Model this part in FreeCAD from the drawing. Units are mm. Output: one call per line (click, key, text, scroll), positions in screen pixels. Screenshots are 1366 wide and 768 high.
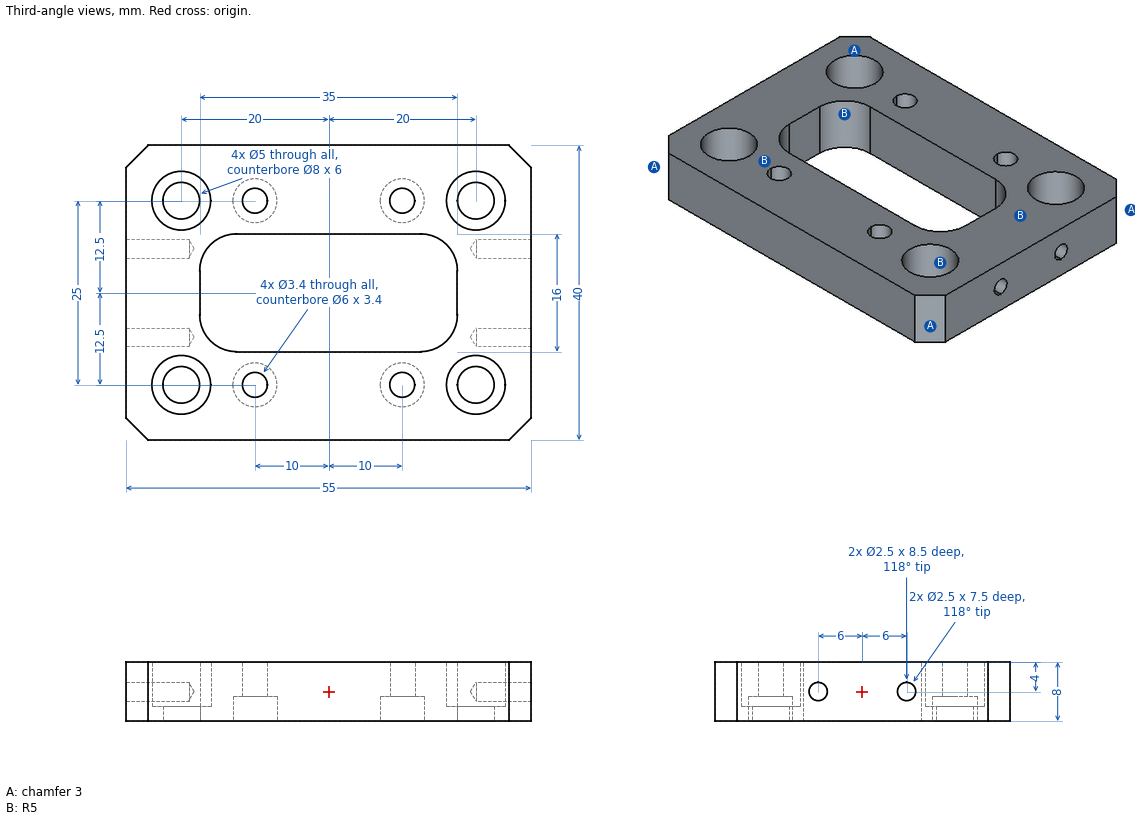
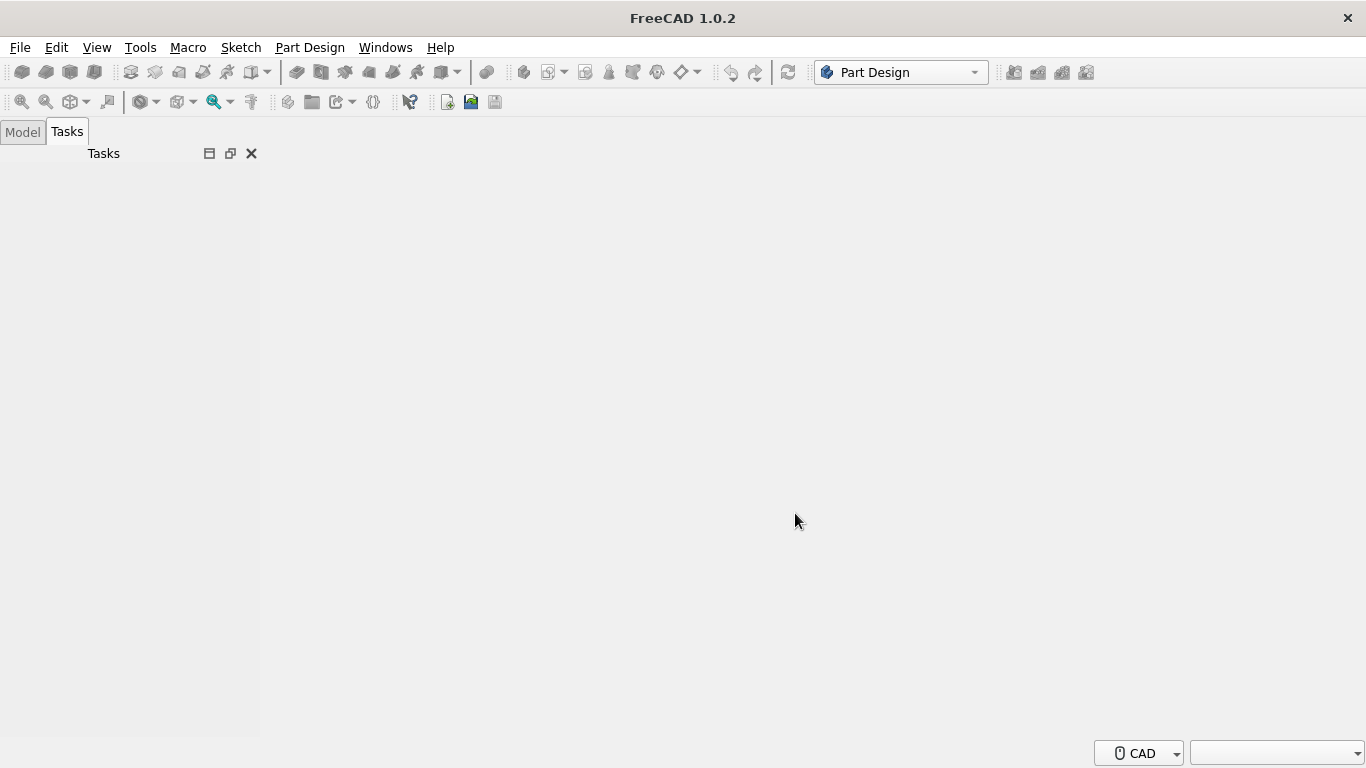
click(448, 102)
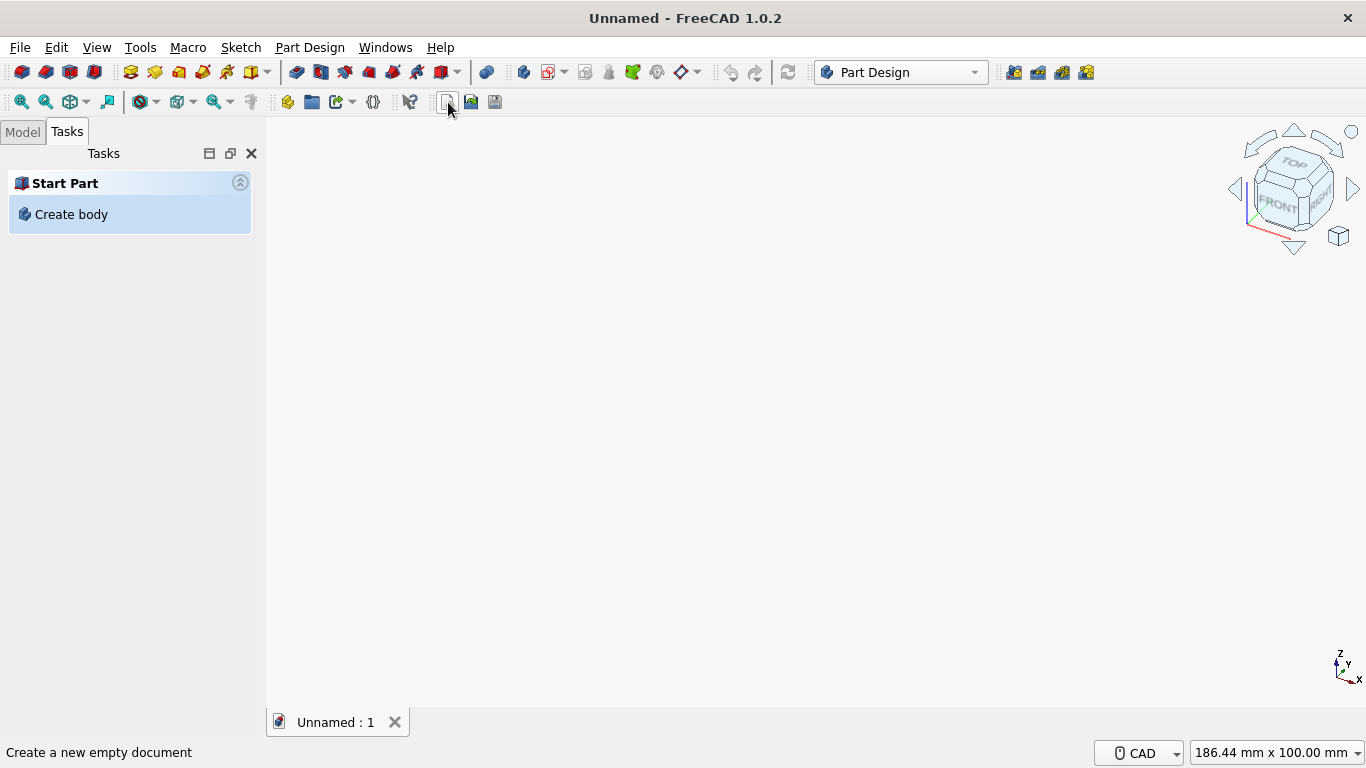
click(524, 72)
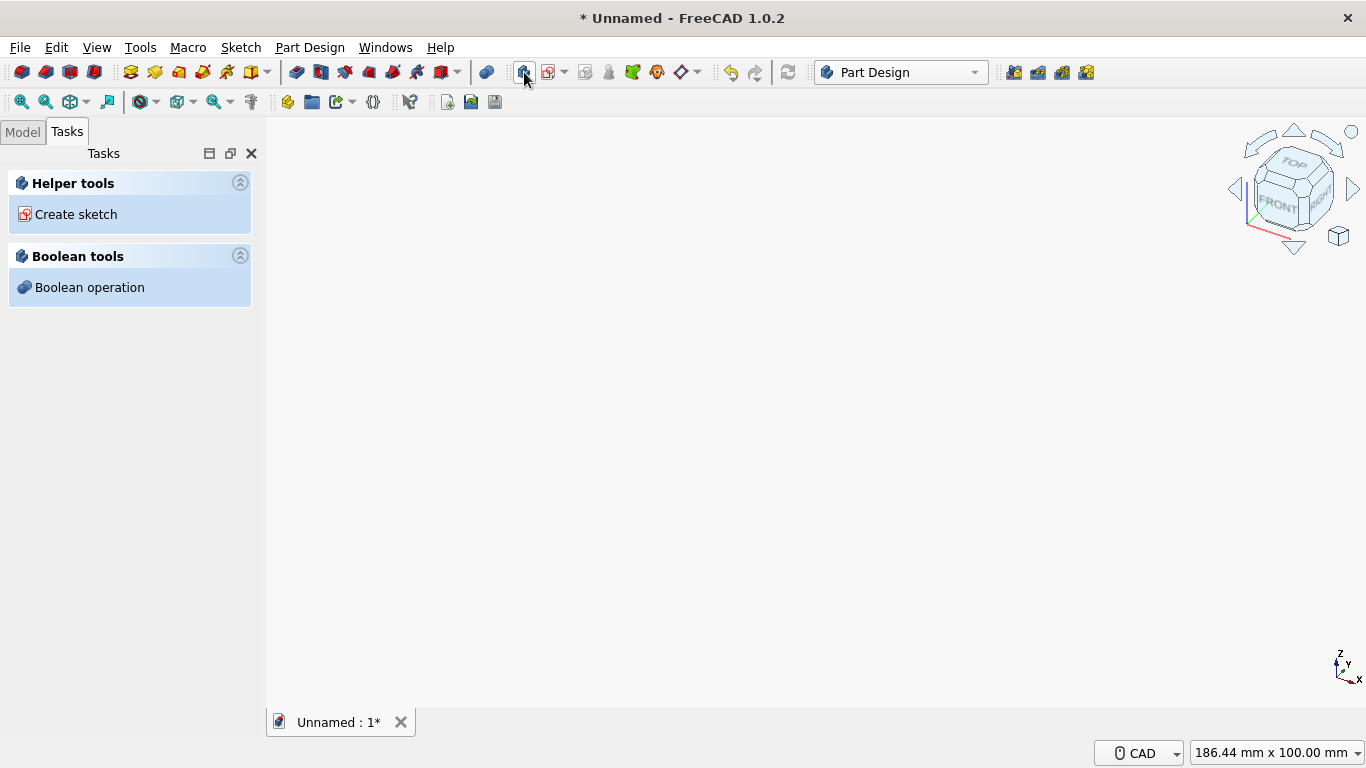
click(23, 131)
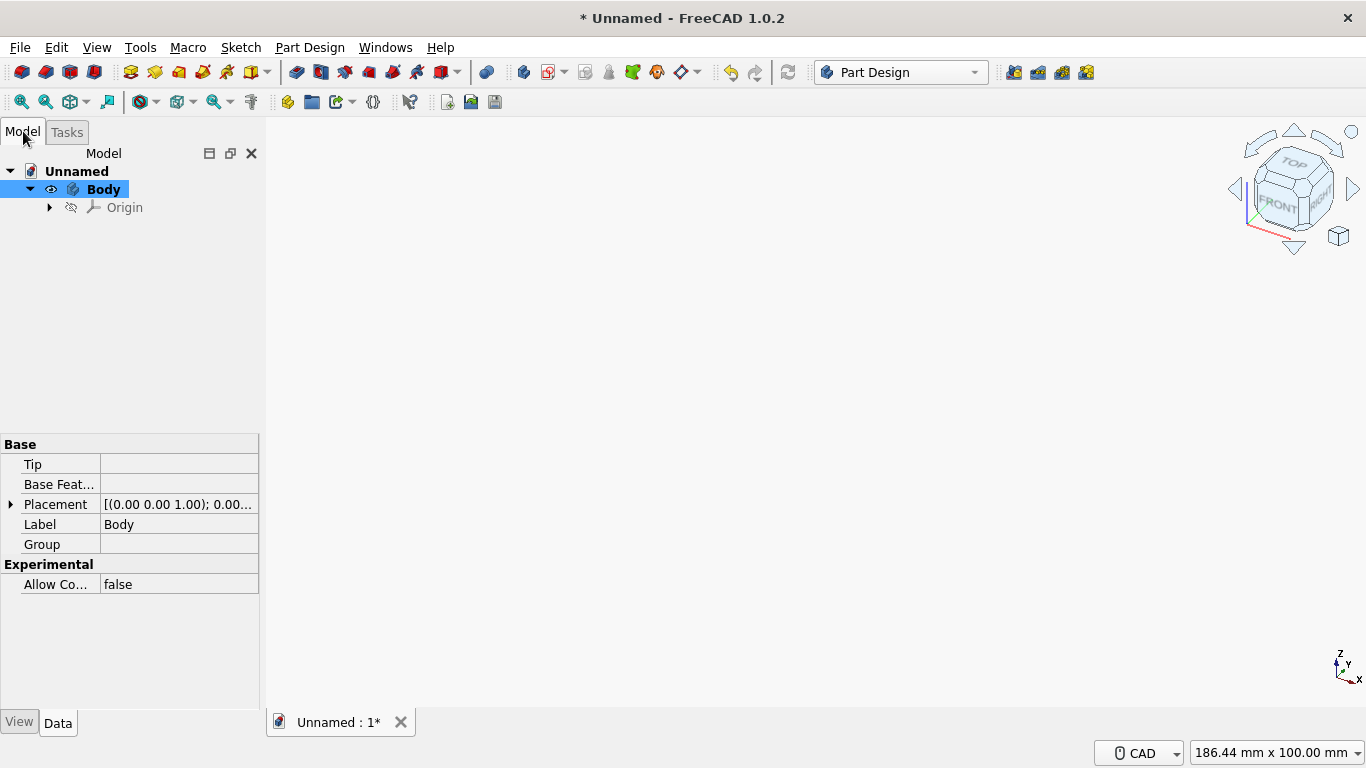
click(50, 207)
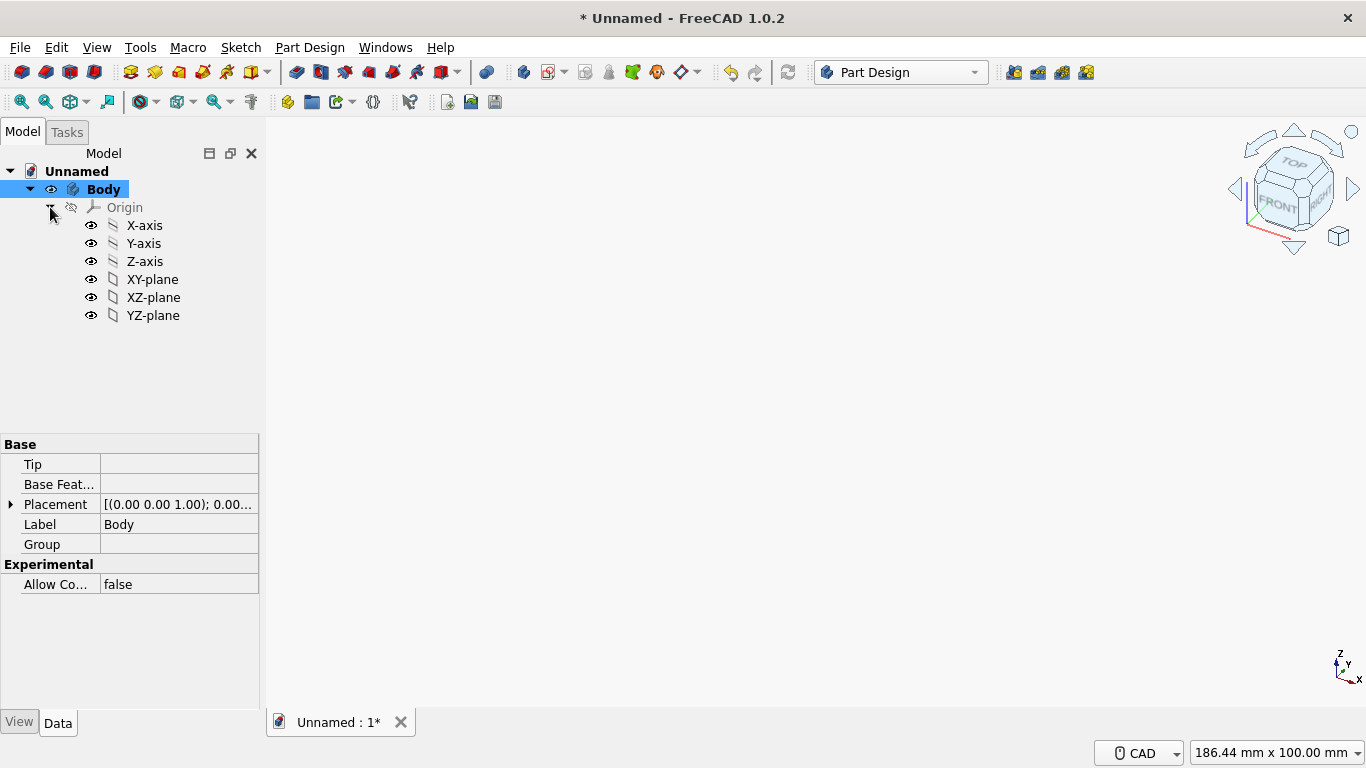
click(136, 279)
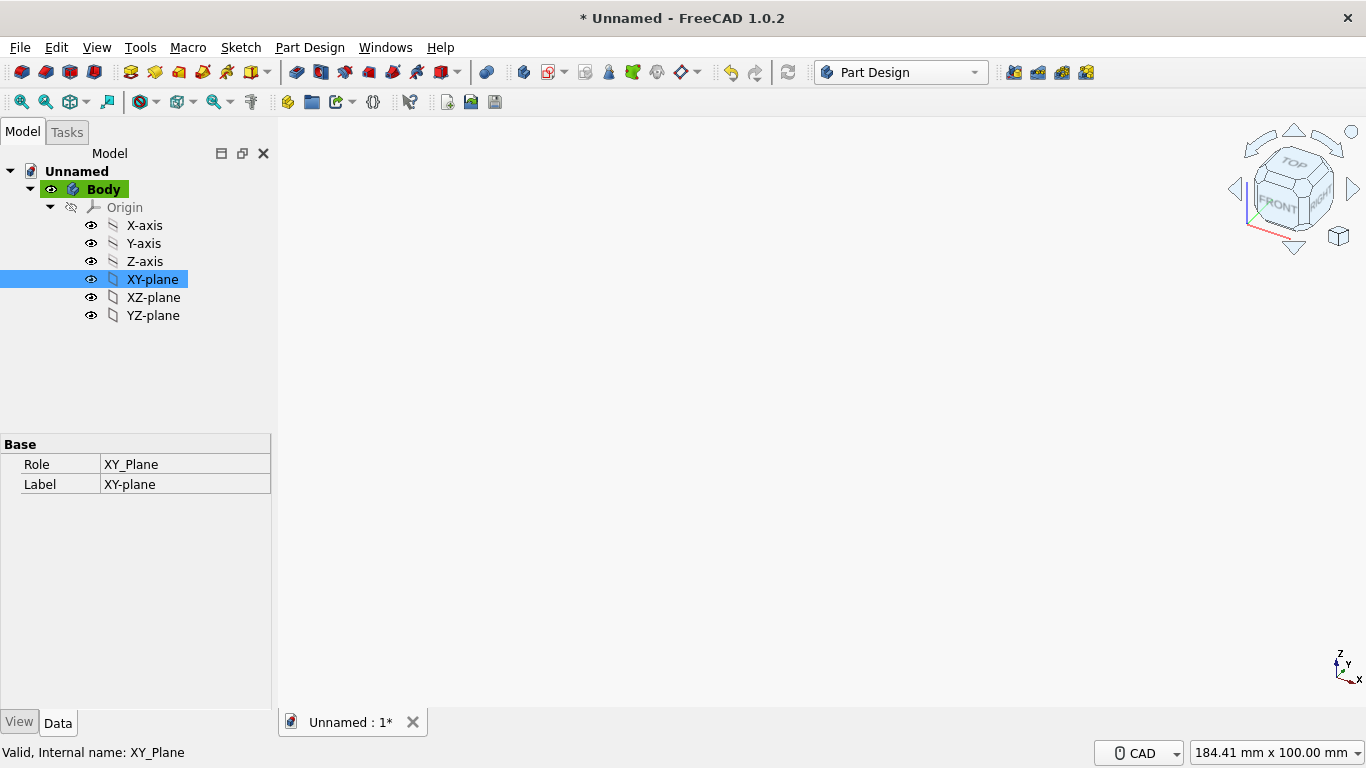
click(682, 72)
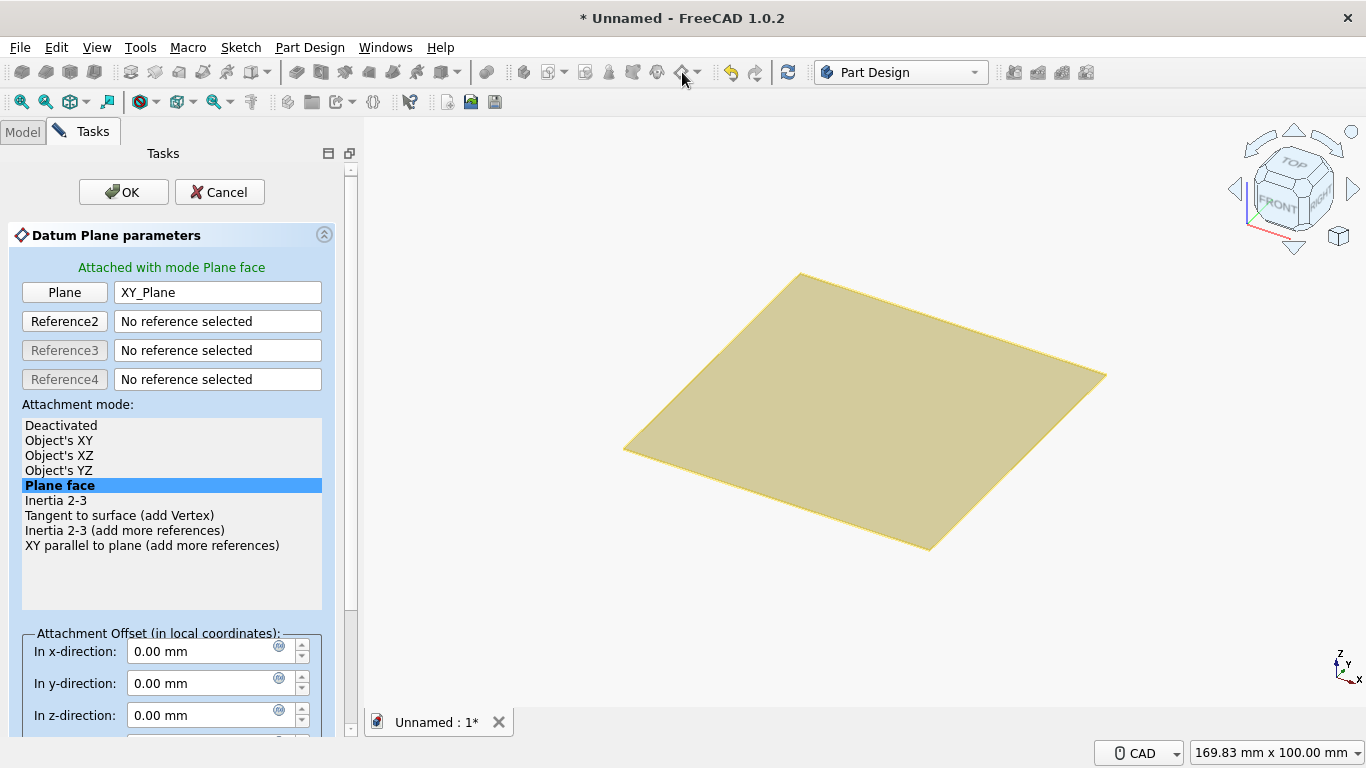
triple_click(210, 715)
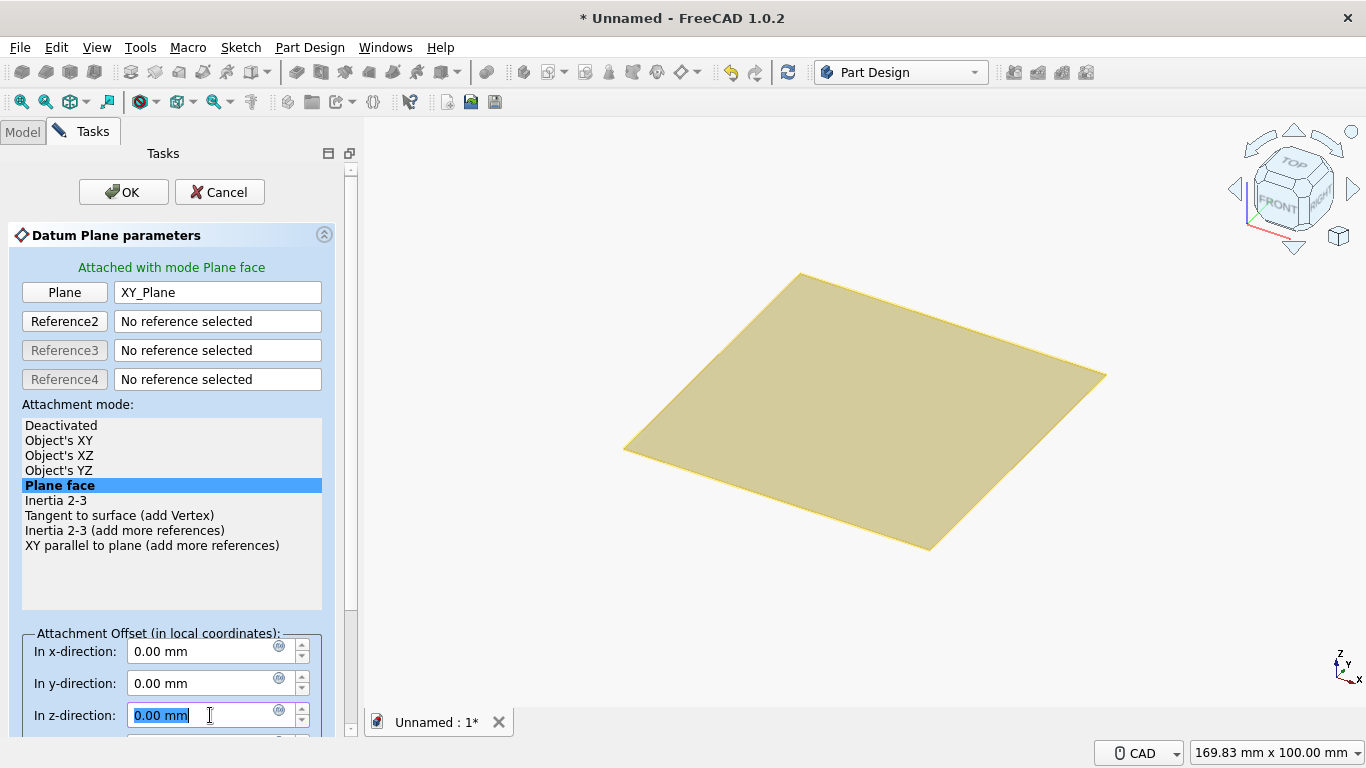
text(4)
key(Tab)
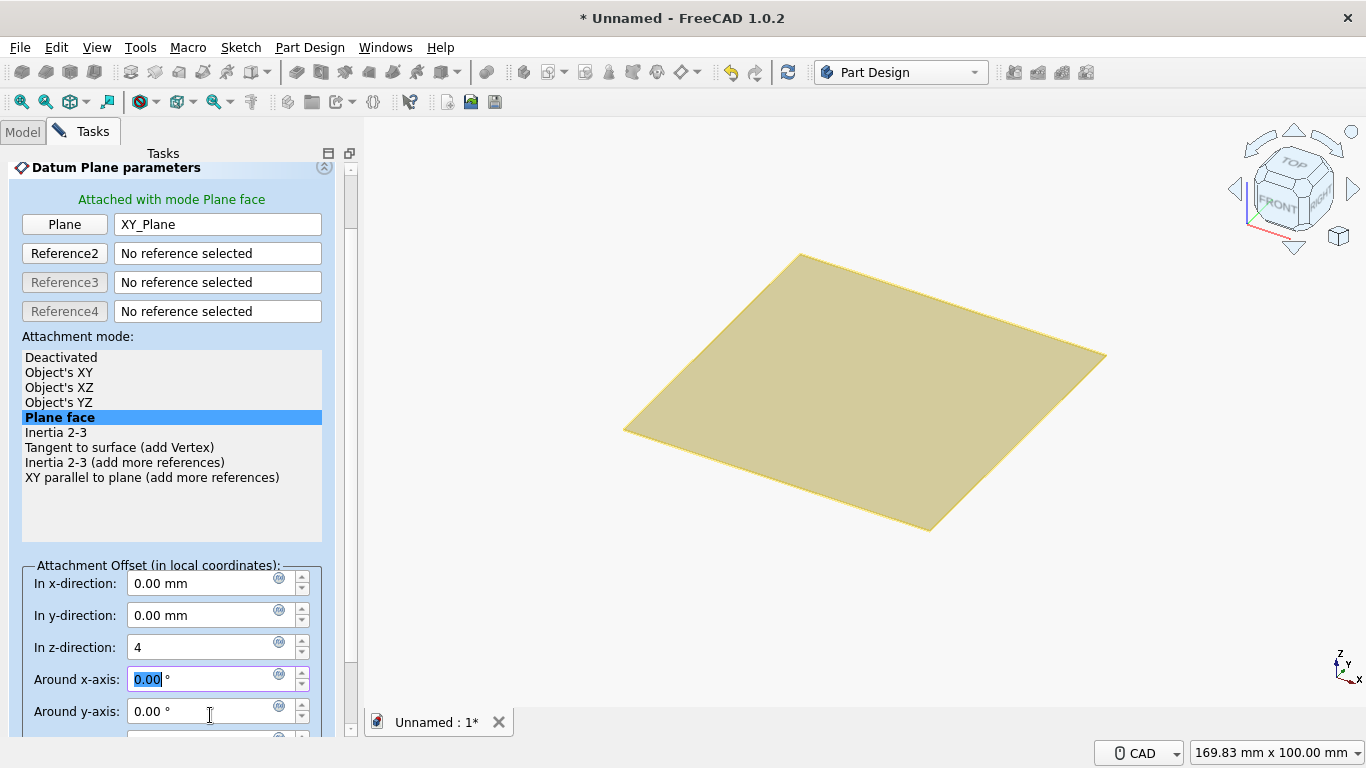
scroll(351, 450, up, 2)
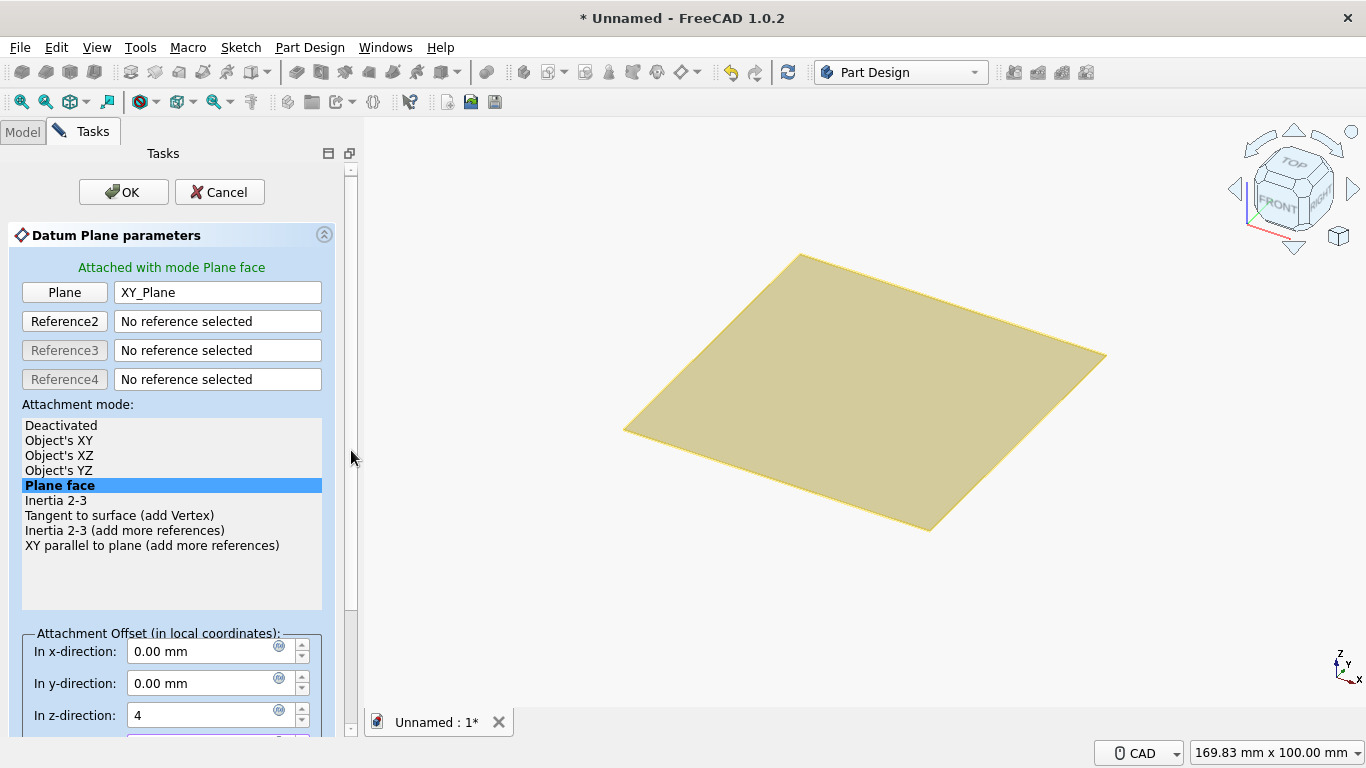
click(124, 192)